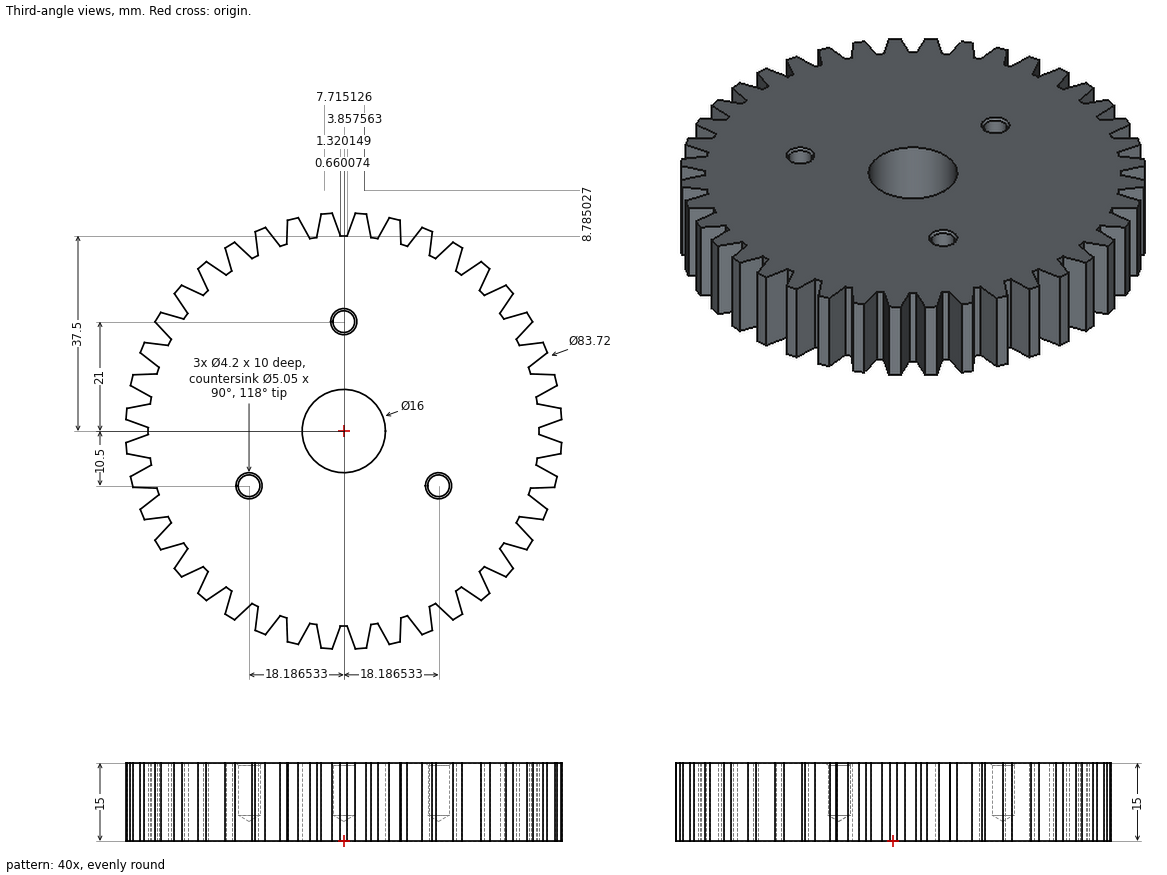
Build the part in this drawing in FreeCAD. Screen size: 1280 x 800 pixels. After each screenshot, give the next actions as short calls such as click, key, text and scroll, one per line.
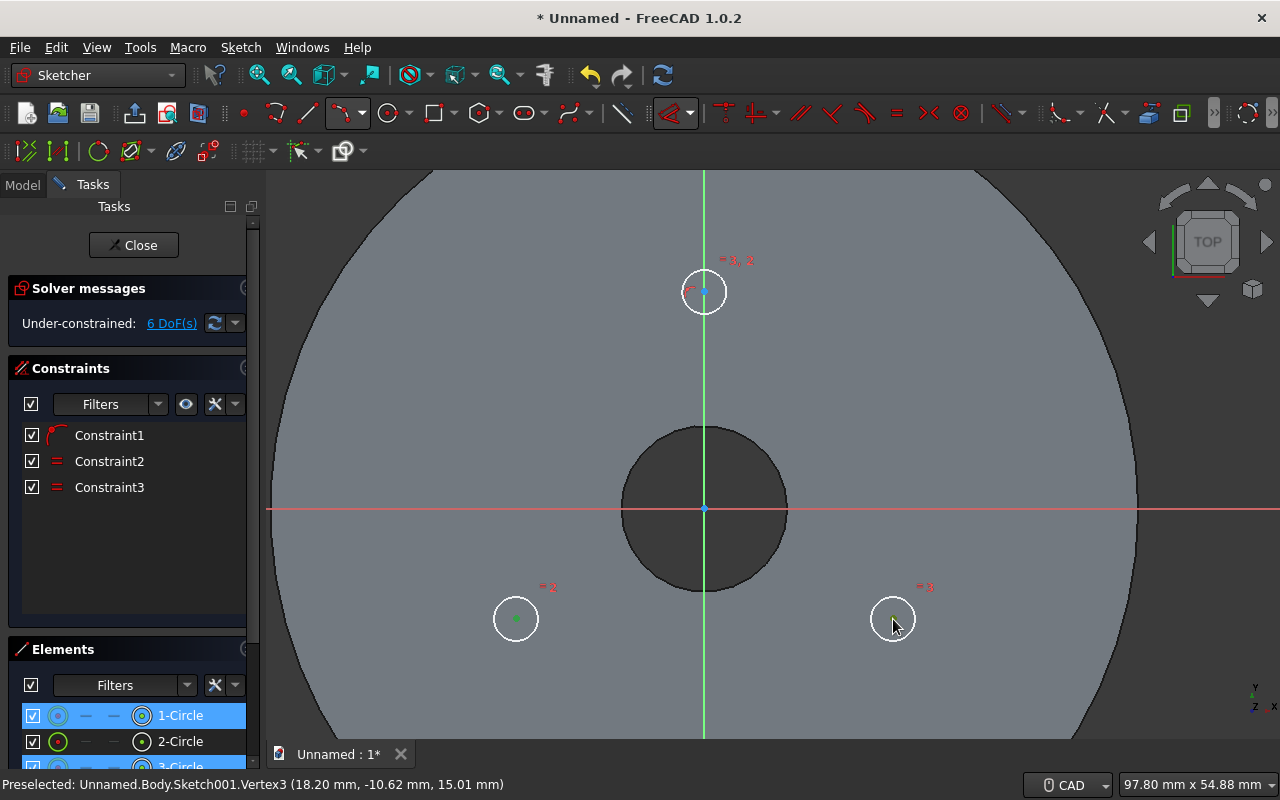
key(h)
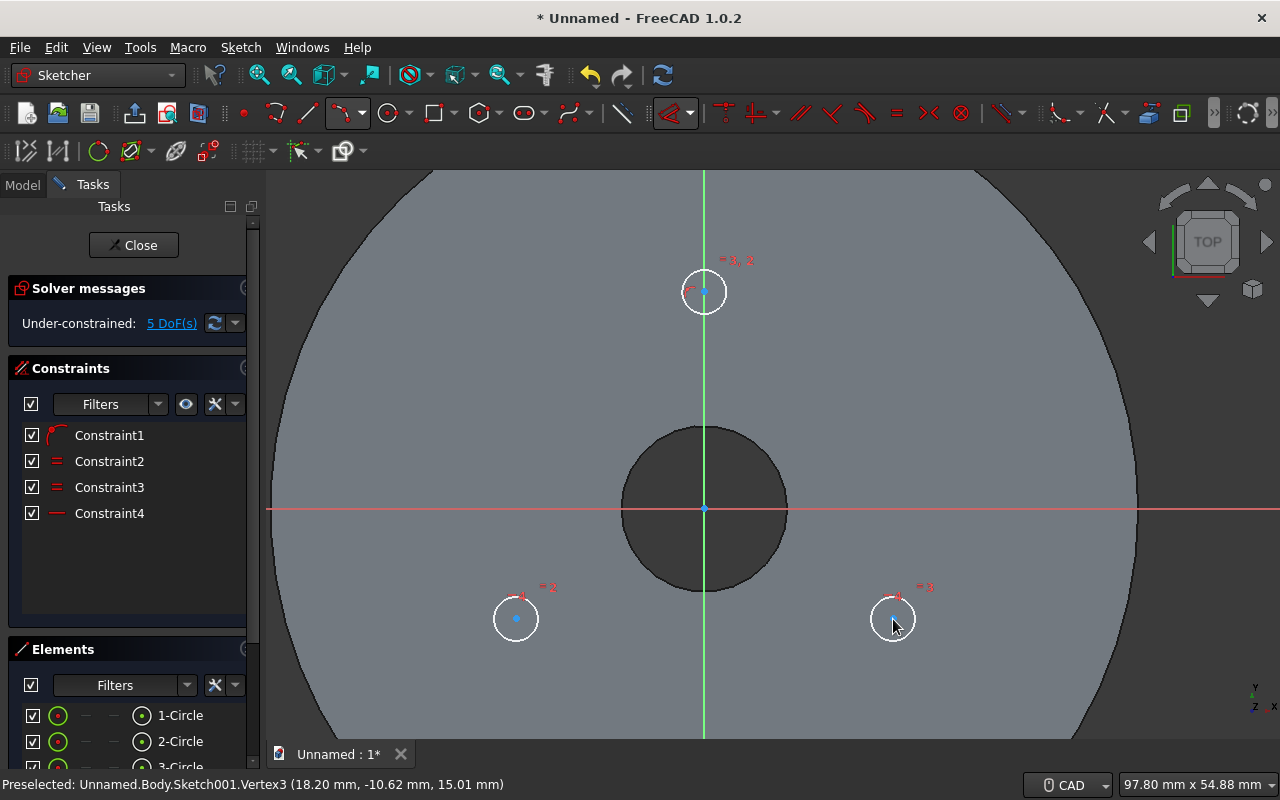
key(d)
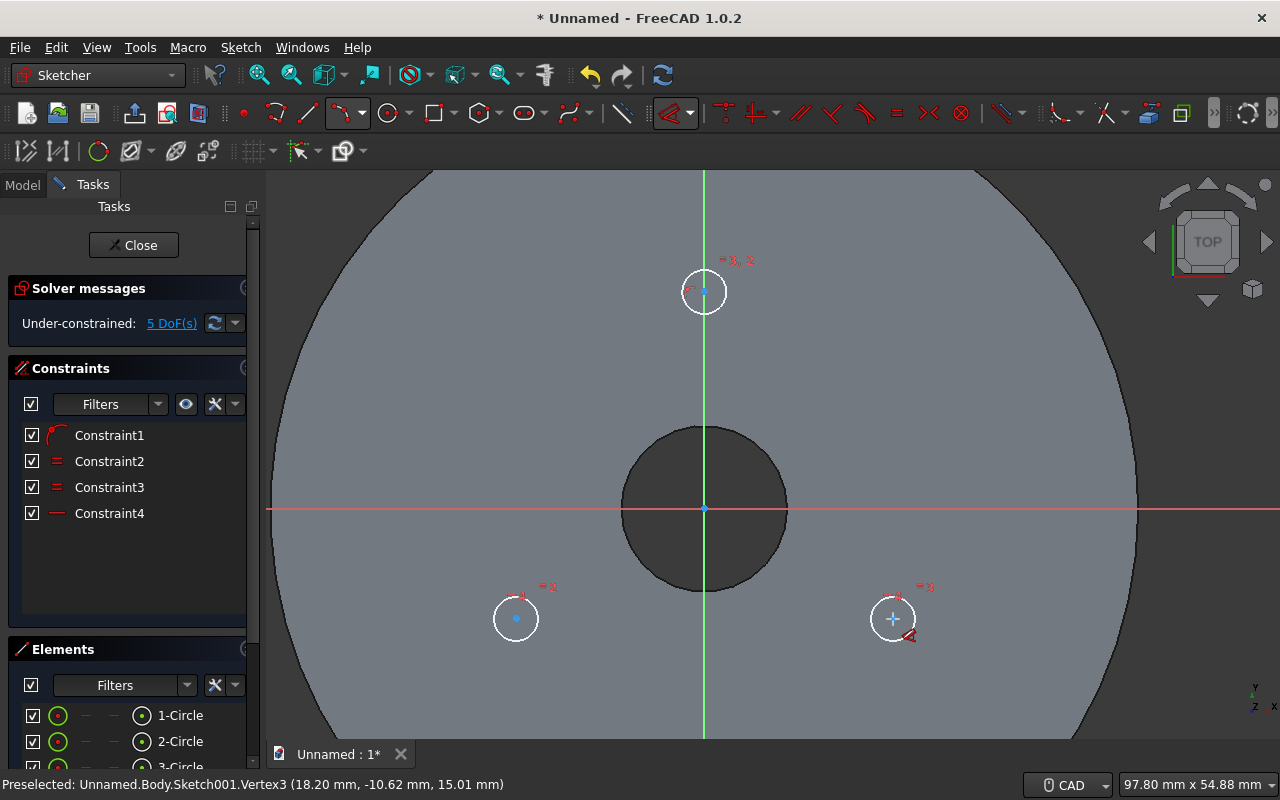
click(531, 603)
click(553, 580)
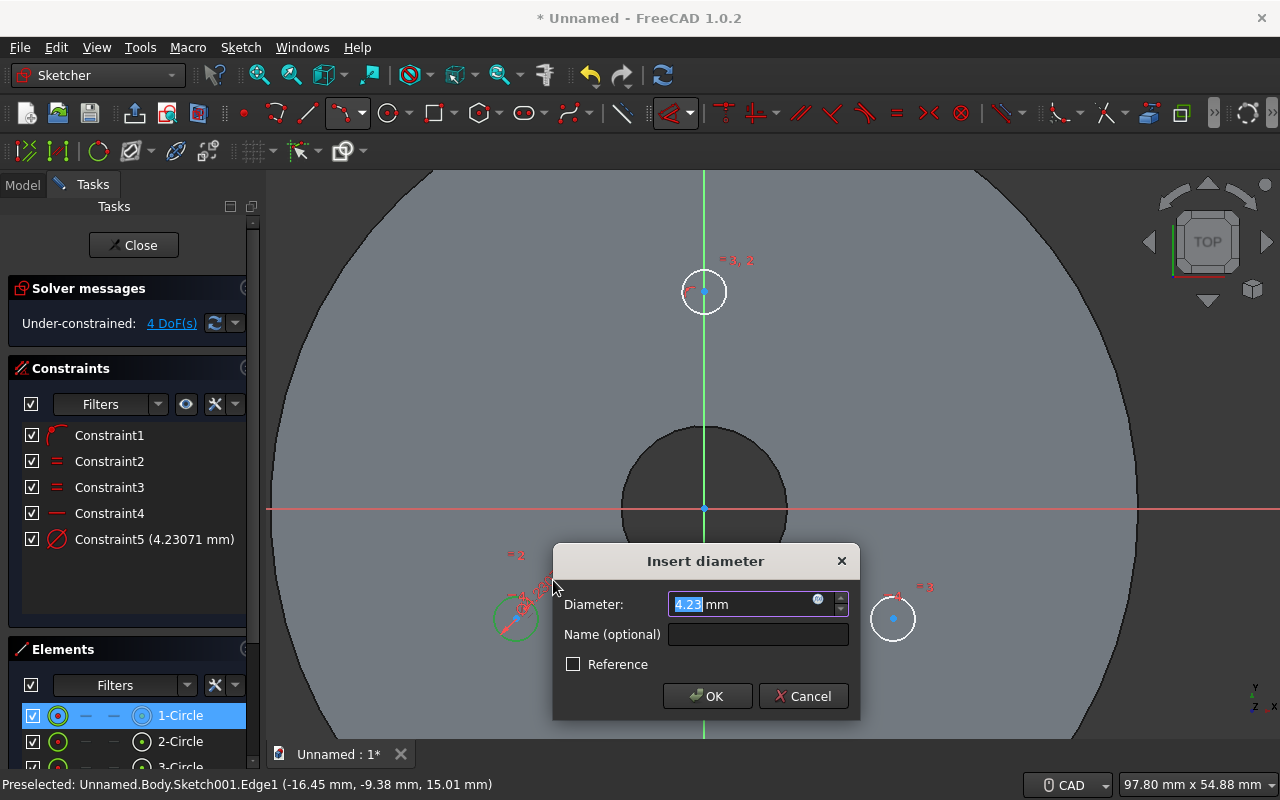
text(4.2)
key(Return)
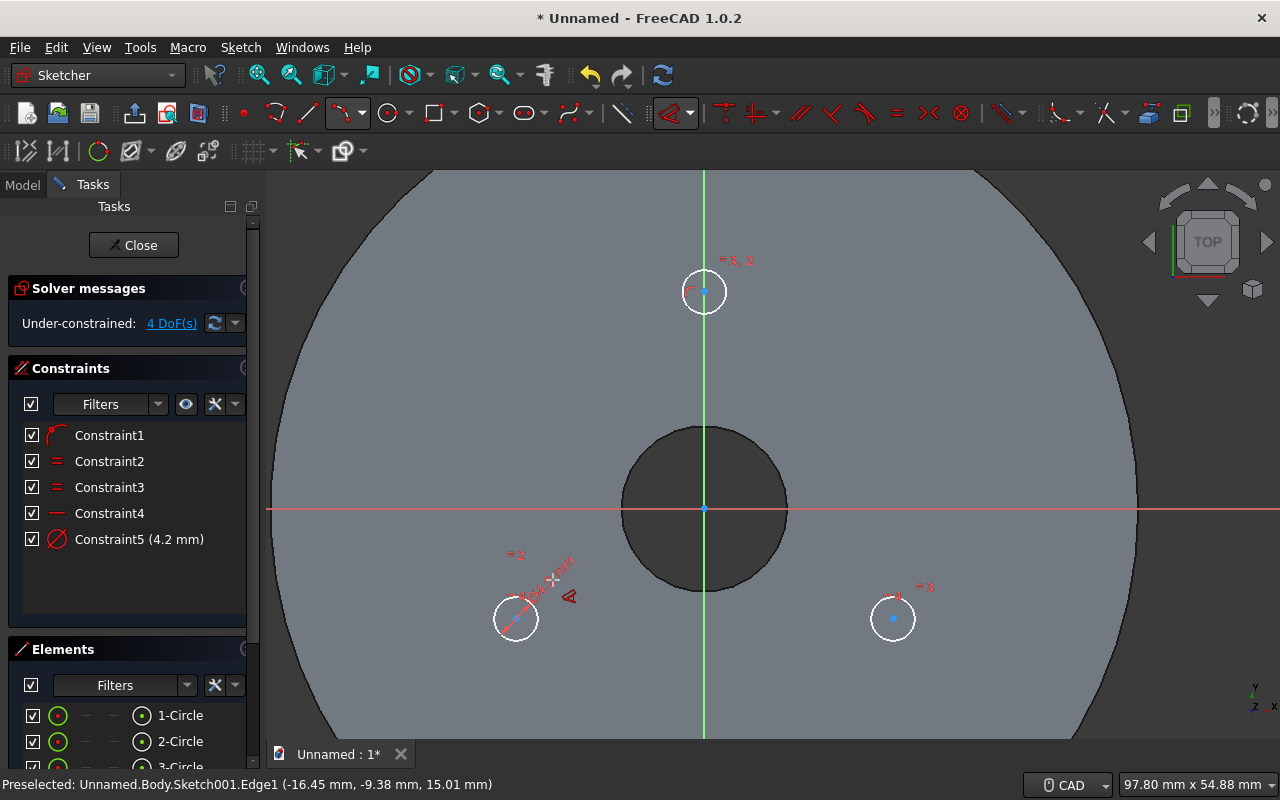
click(704, 292)
click(738, 400)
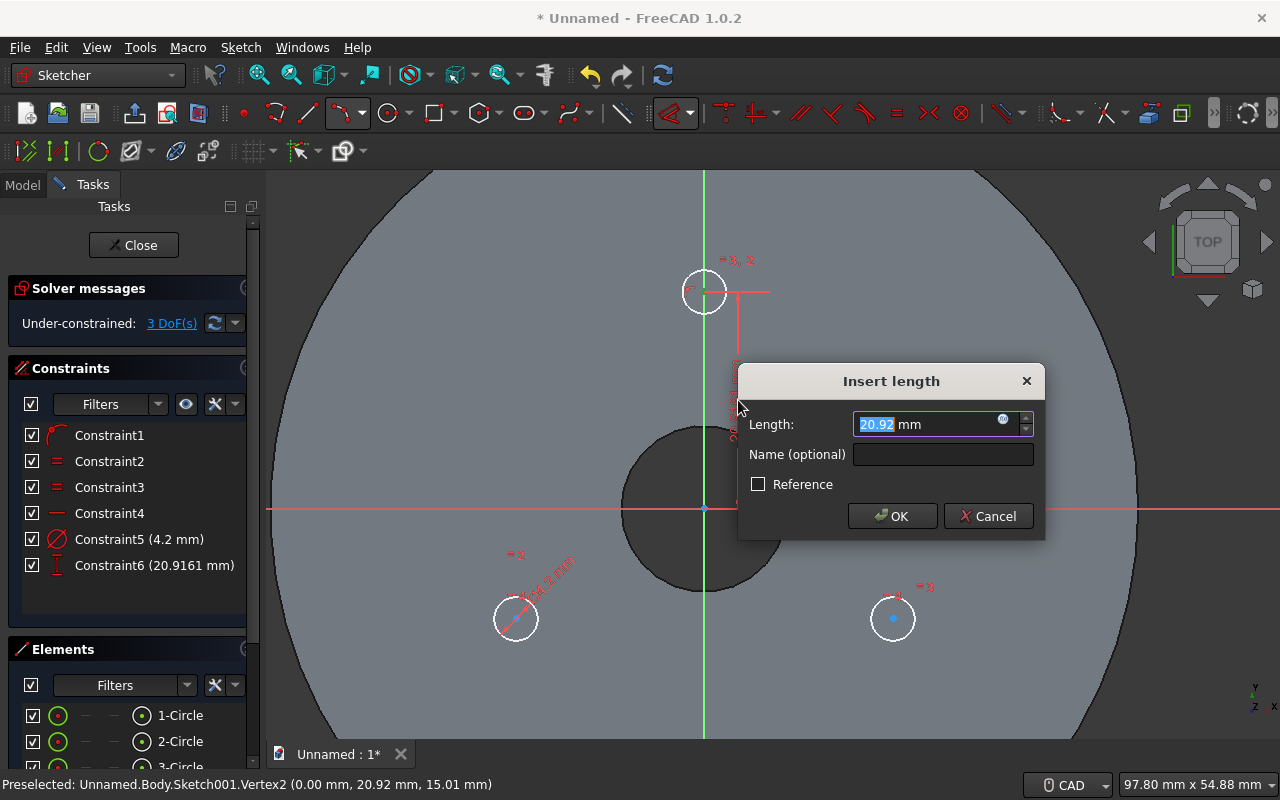
text(21)
key(Return)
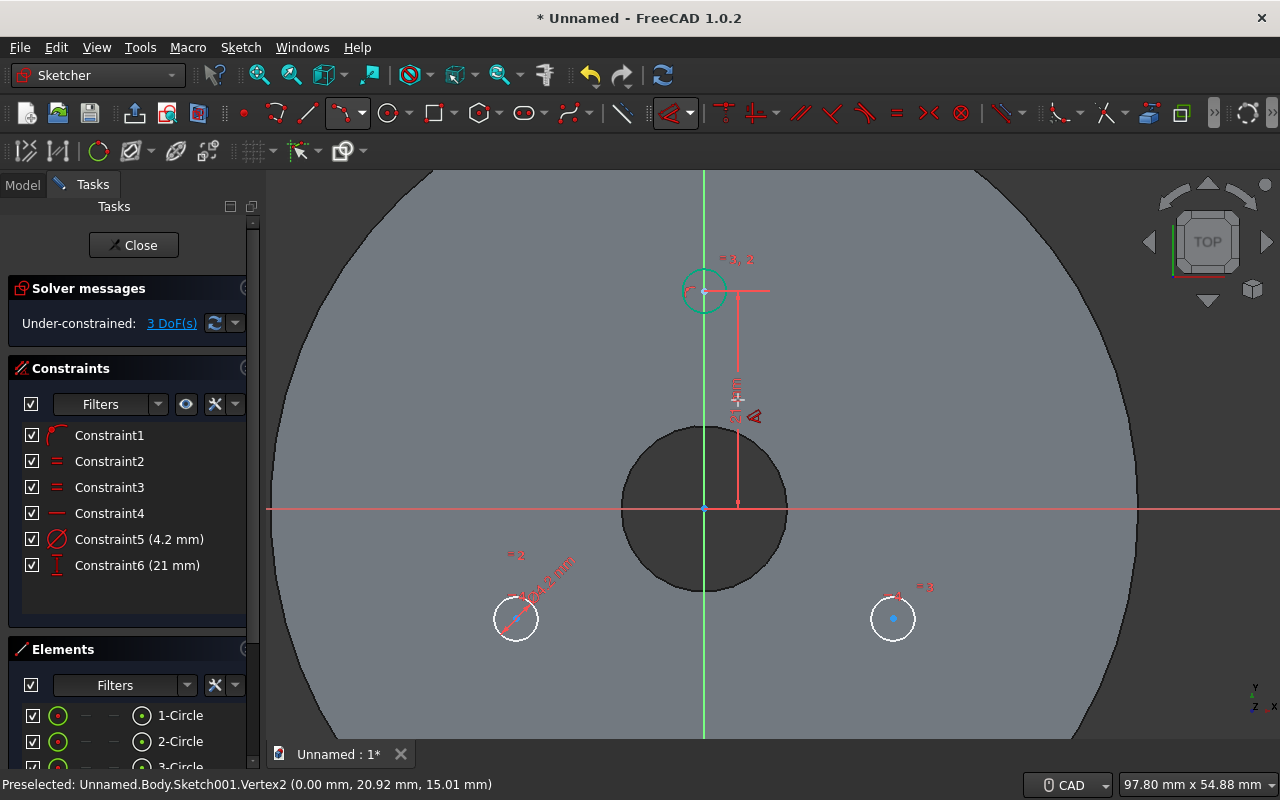
click(516, 619)
click(482, 564)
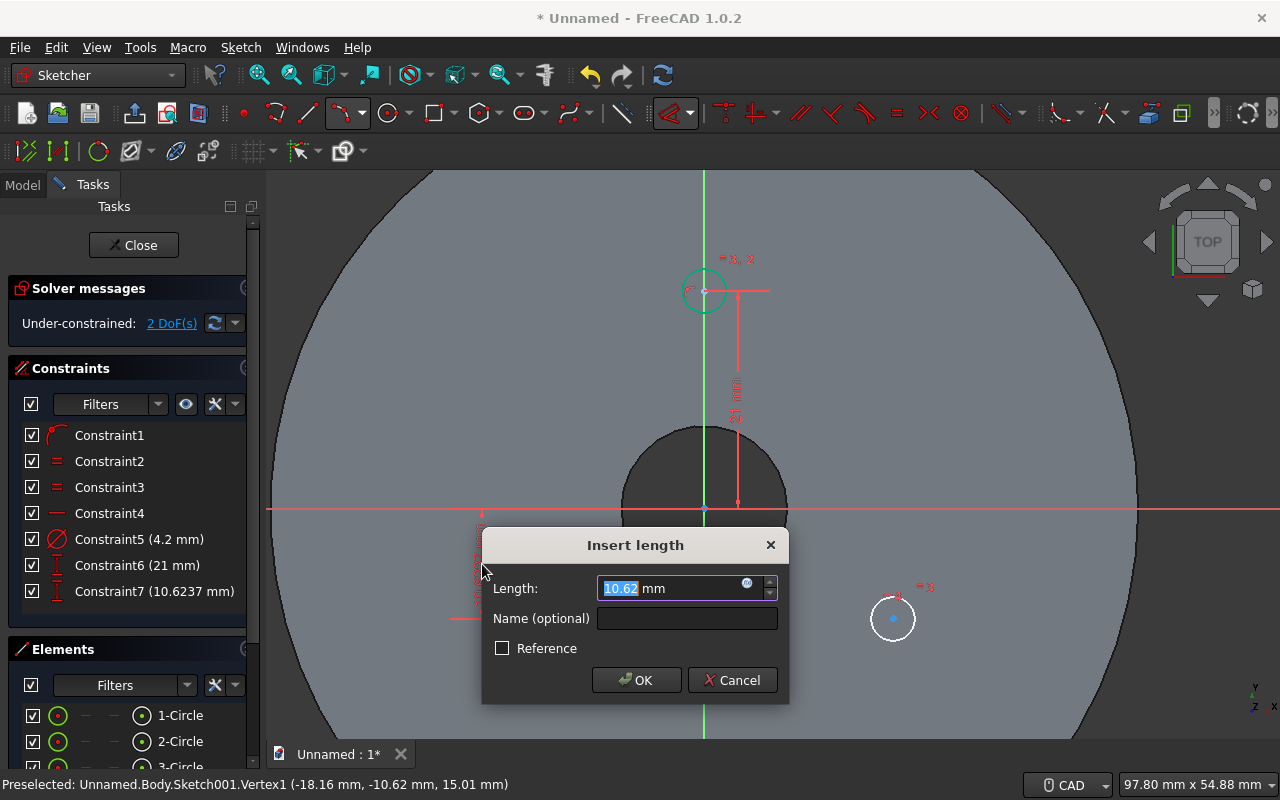
text(10.5)
key(Return)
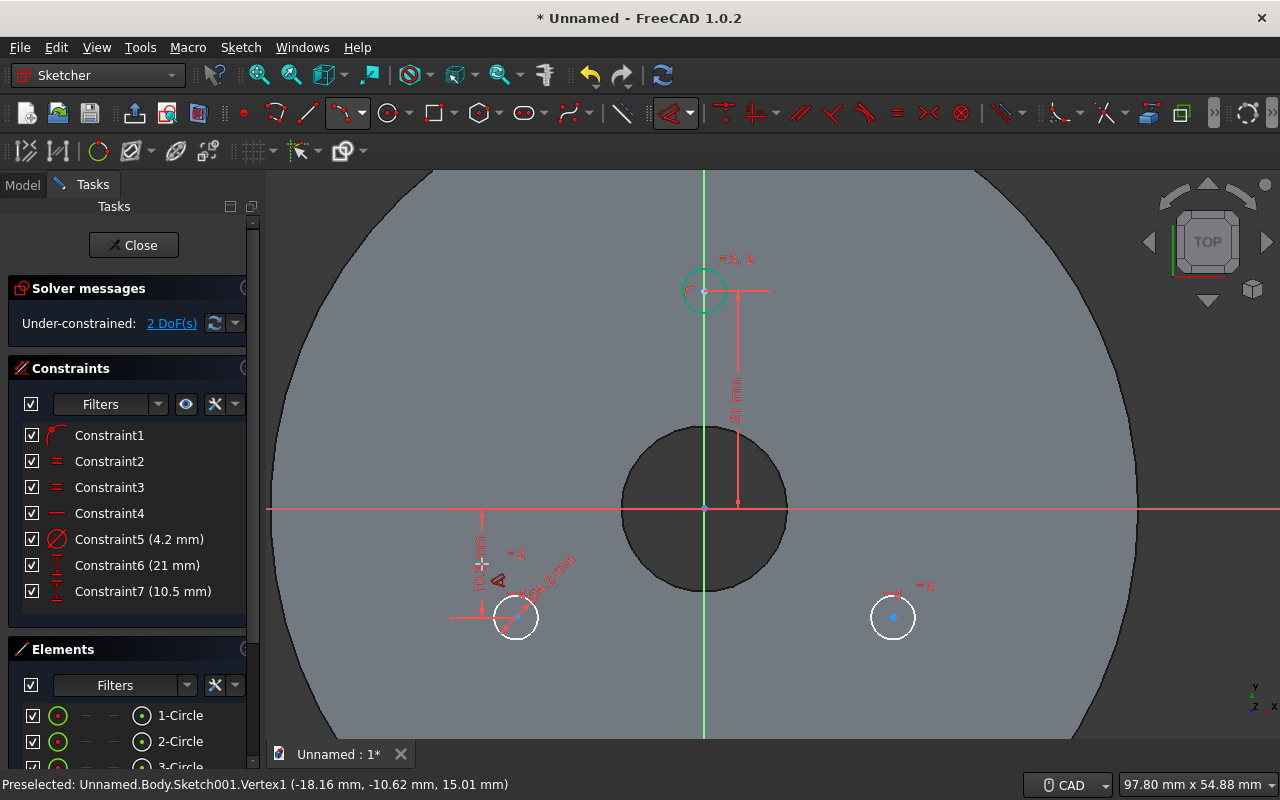
click(516, 618)
click(610, 652)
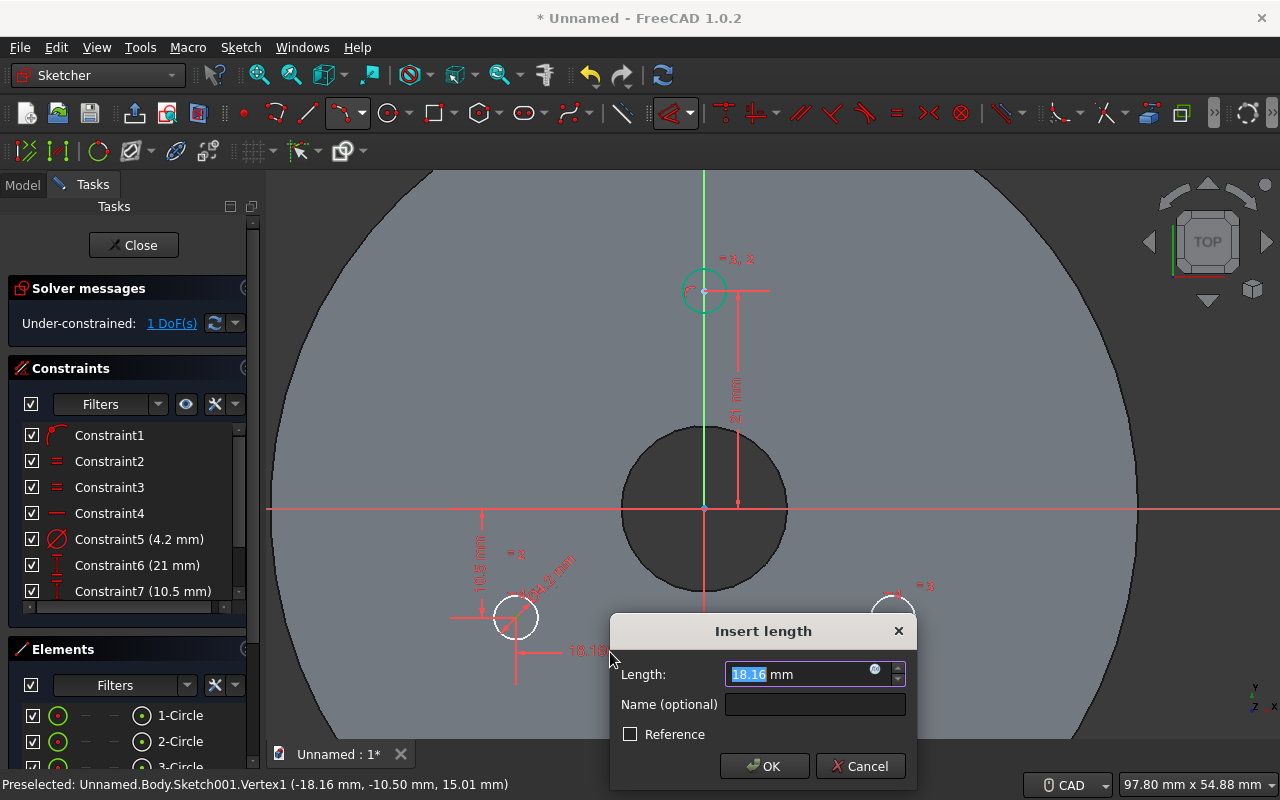
text(18.186533)
key(Return)